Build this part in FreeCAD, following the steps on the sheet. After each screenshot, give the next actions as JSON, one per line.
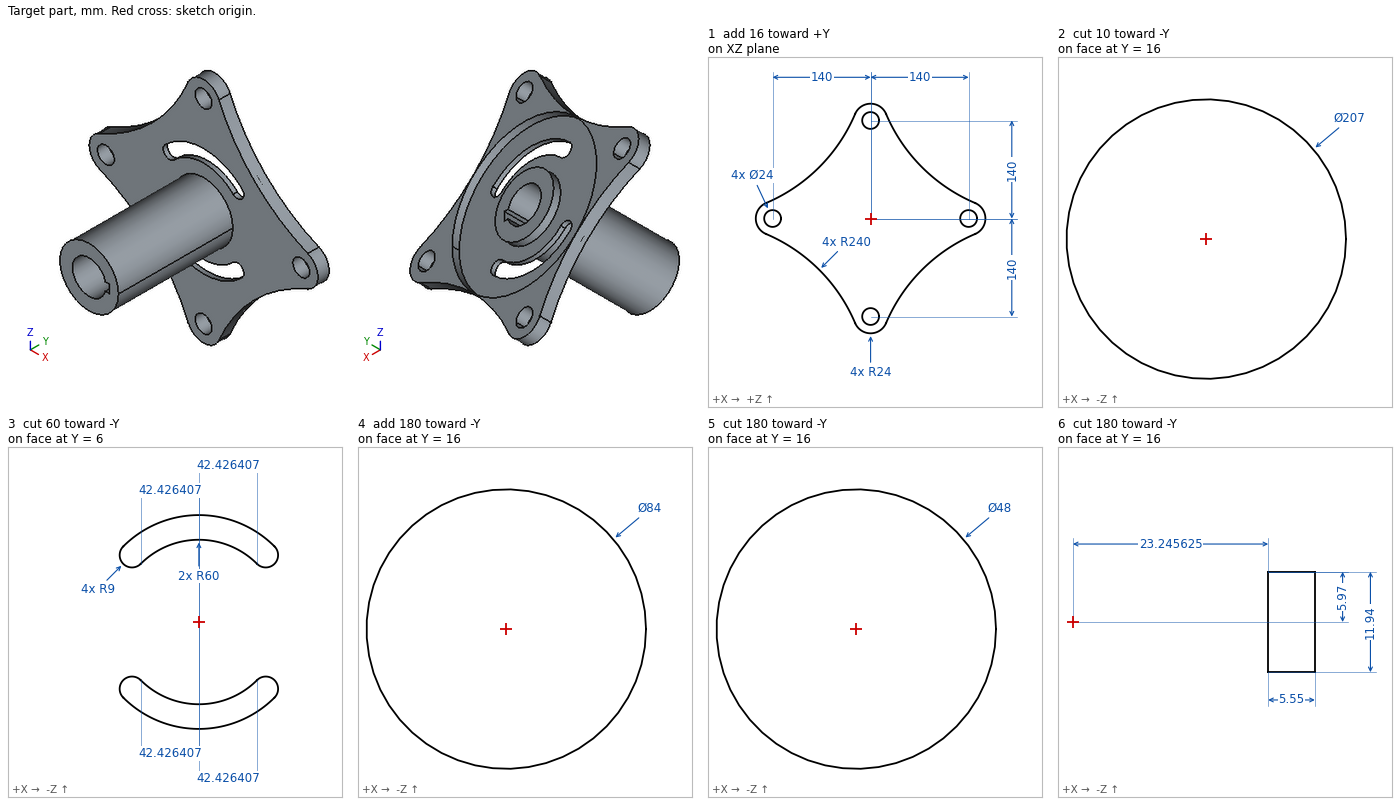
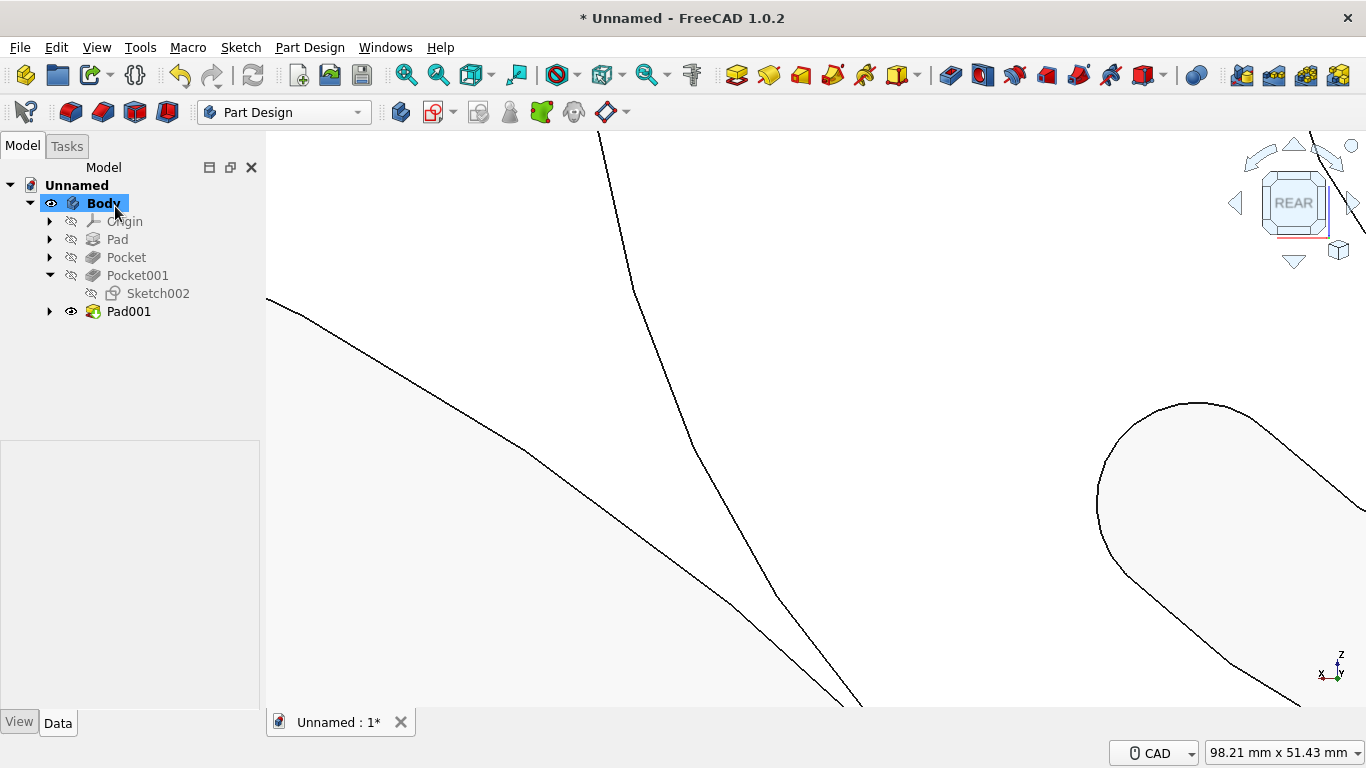
{"action": "left_click", "coordinate": [408, 76]}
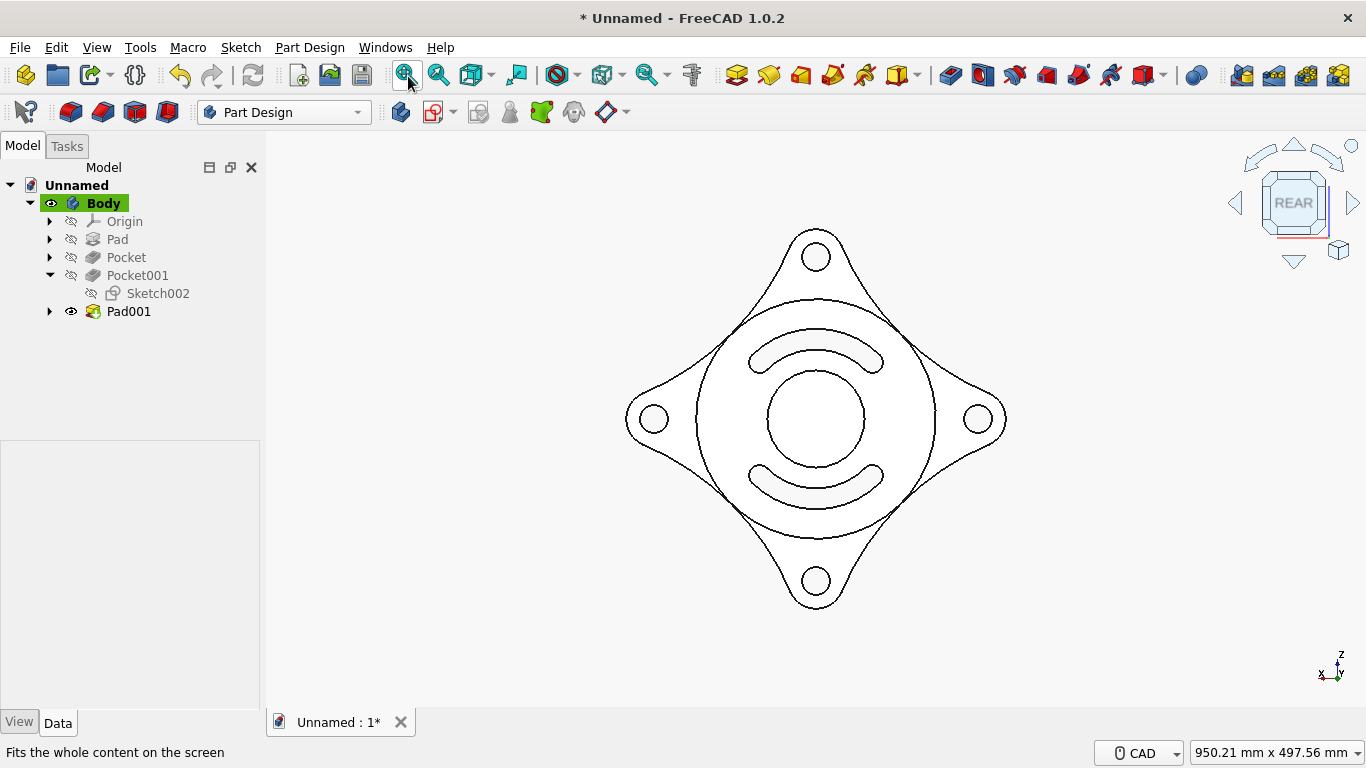
{"action": "scroll", "coordinate": [708, 472], "scroll_direction": "up", "scroll_amount": 11}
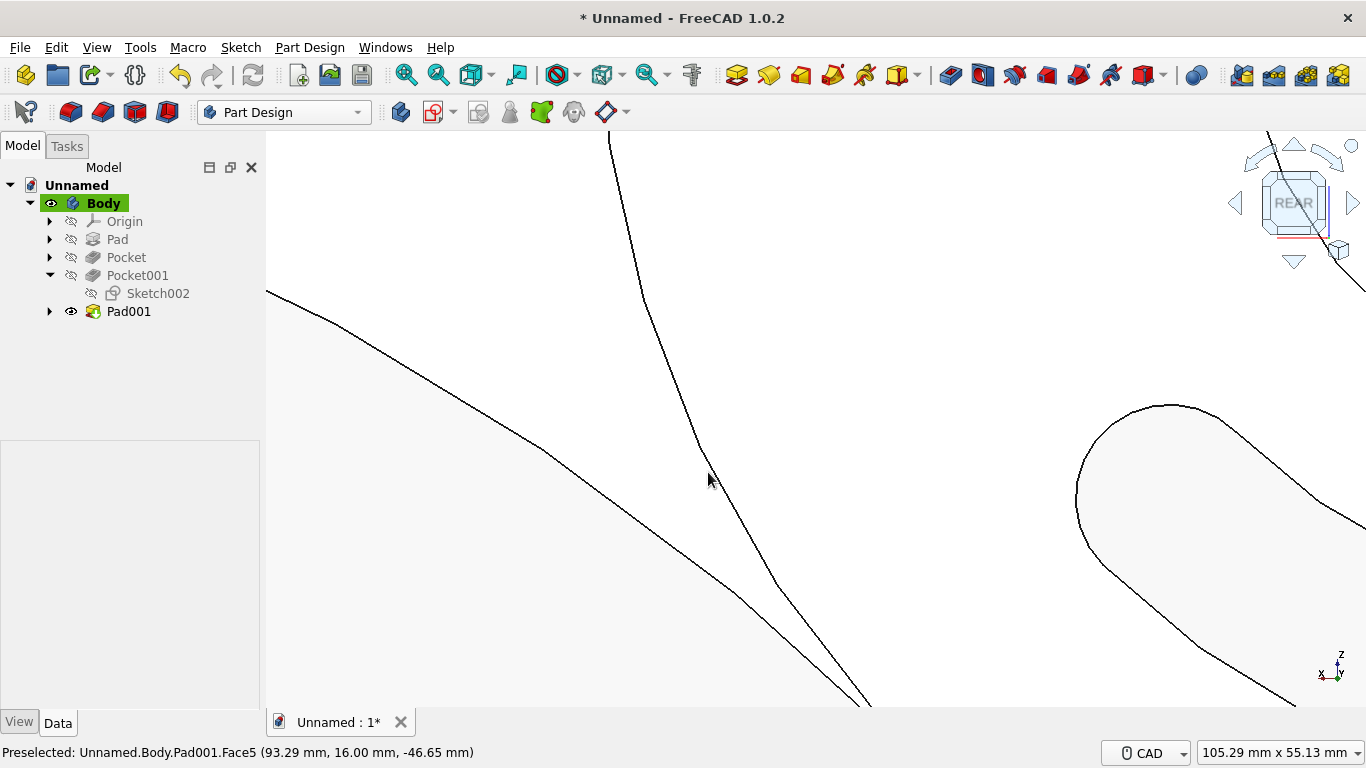
{"action": "left_click", "coordinate": [700, 477]}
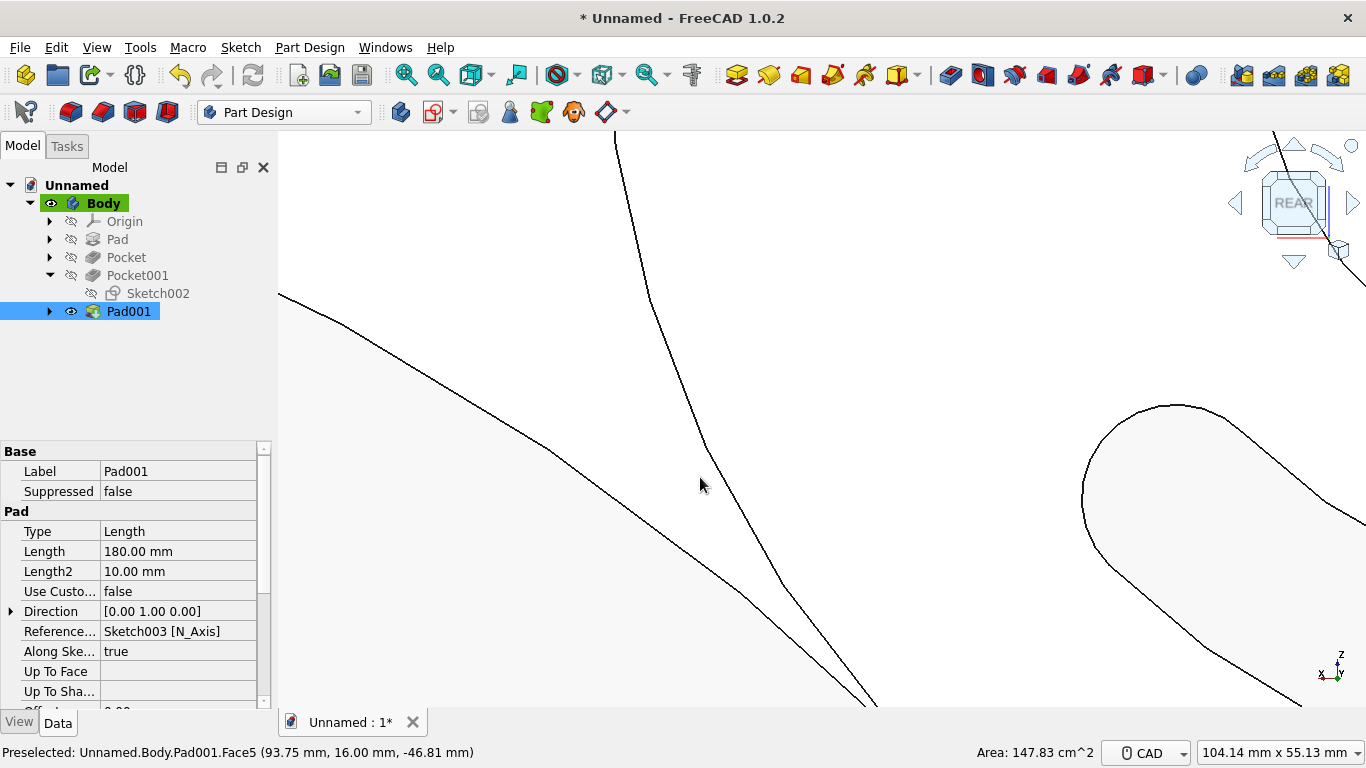
{"action": "left_click", "coordinate": [434, 112]}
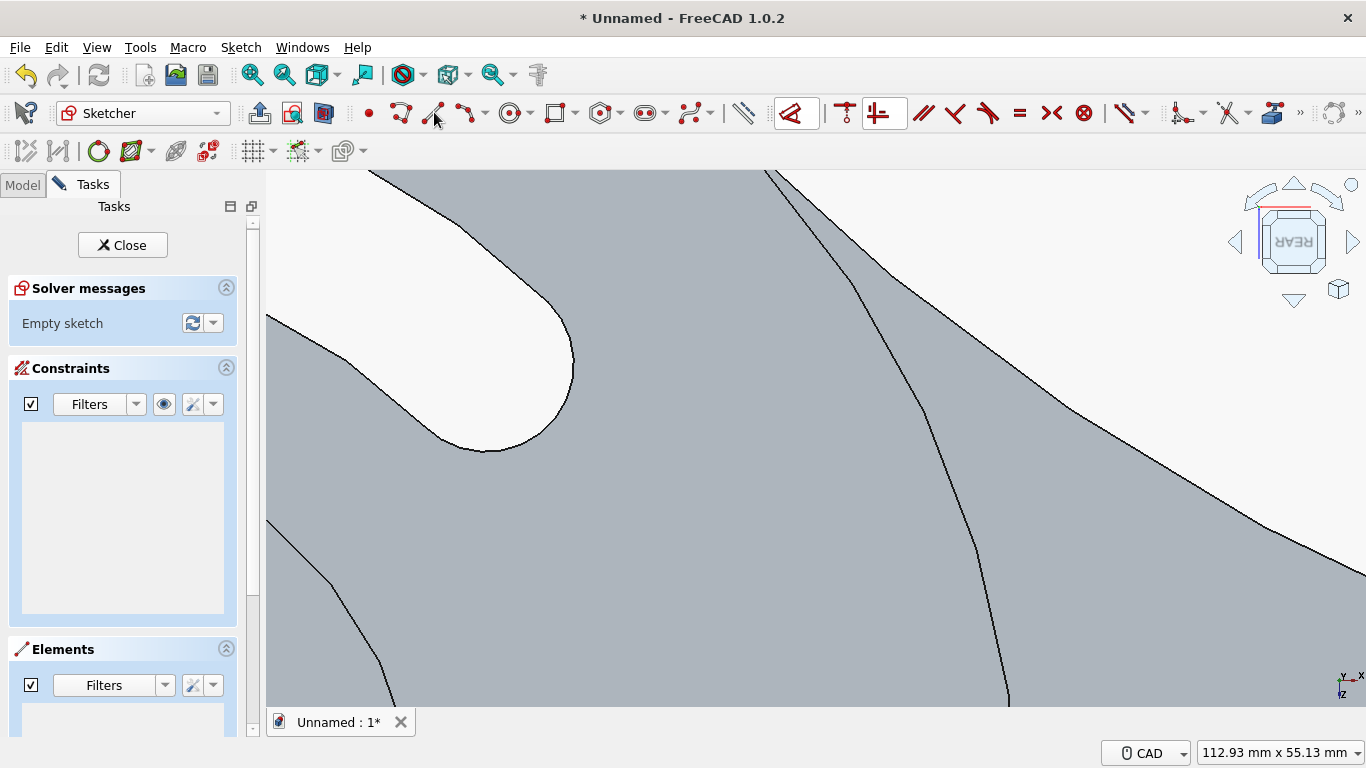
{"action": "scroll", "coordinate": [1201, 198], "scroll_direction": "down", "scroll_amount": 4}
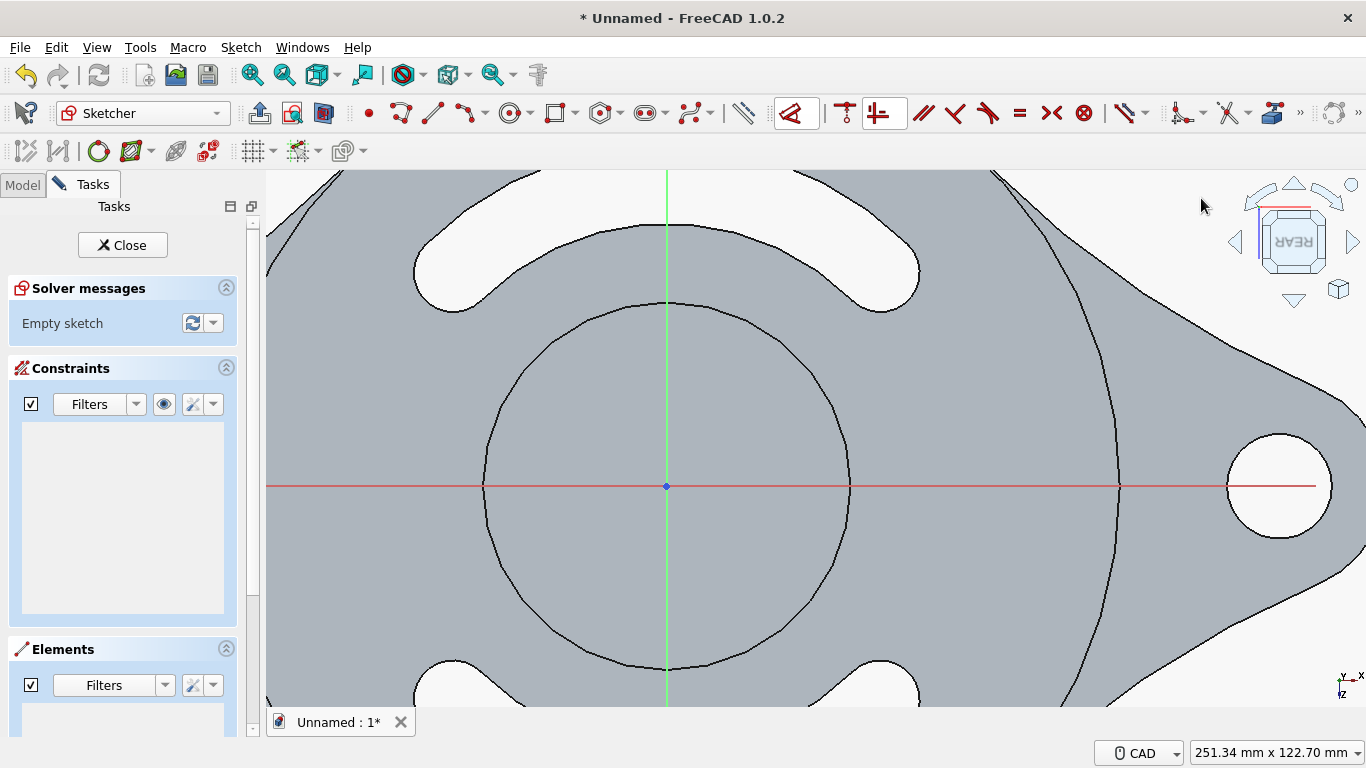
{"action": "scroll", "coordinate": [503, 583], "scroll_direction": "up", "scroll_amount": 2}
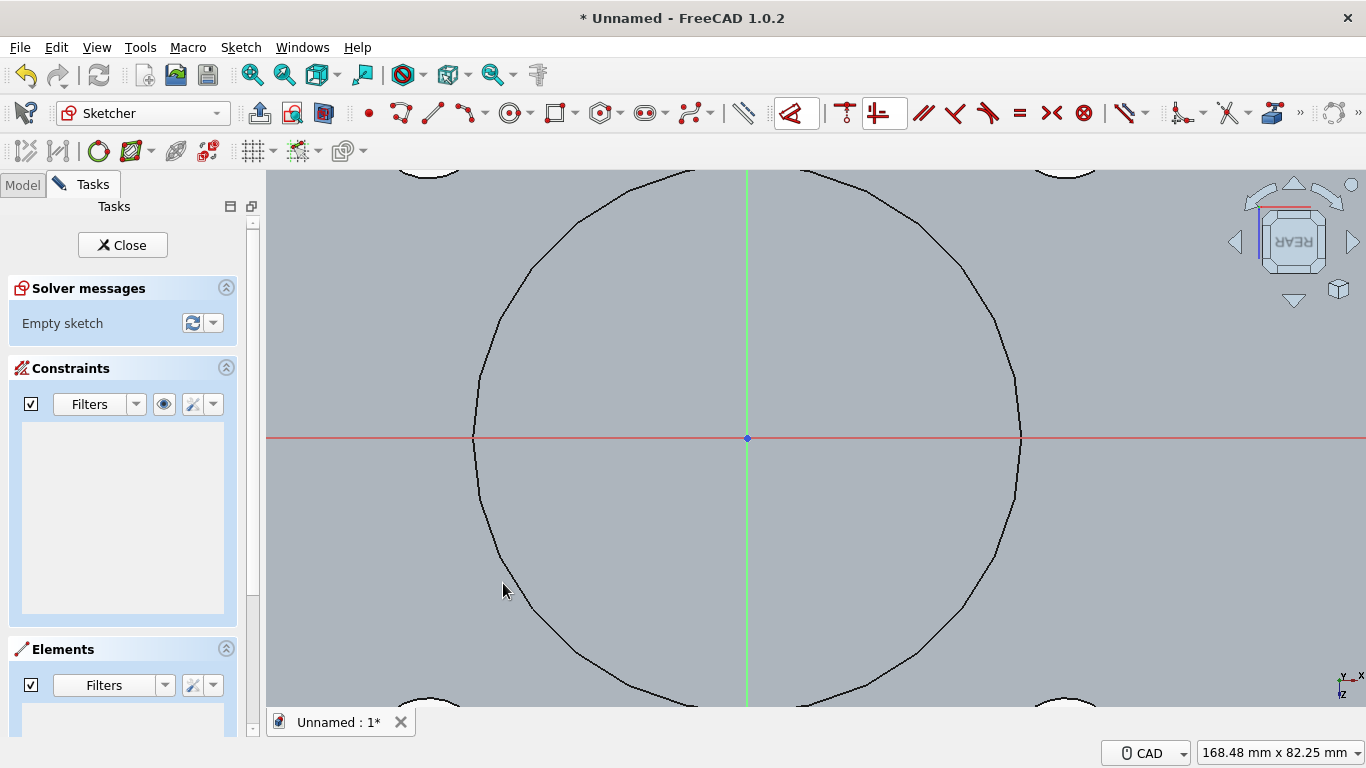
{"action": "left_click", "coordinate": [510, 114]}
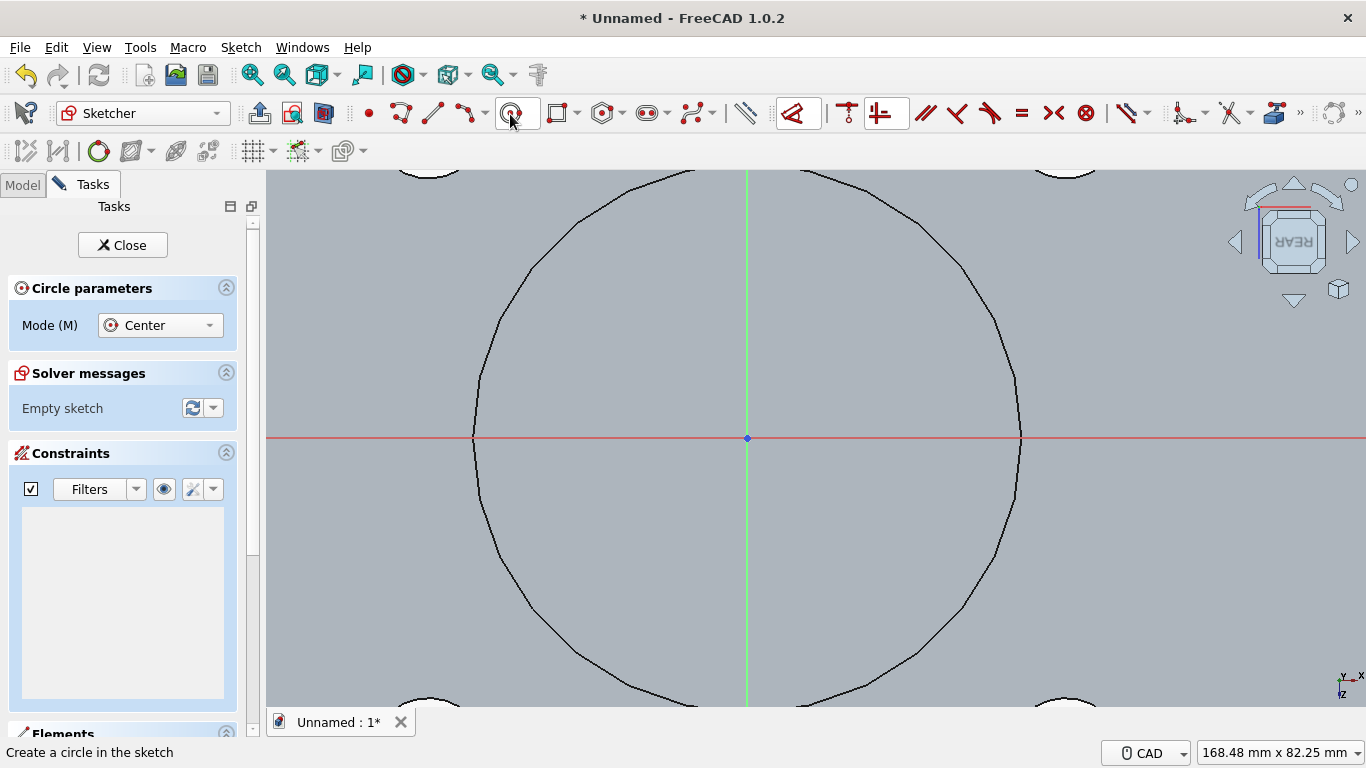
{"action": "left_click", "coordinate": [747, 438]}
{"action": "left_click", "coordinate": [858, 327]}
{"action": "key", "text": "Escape"}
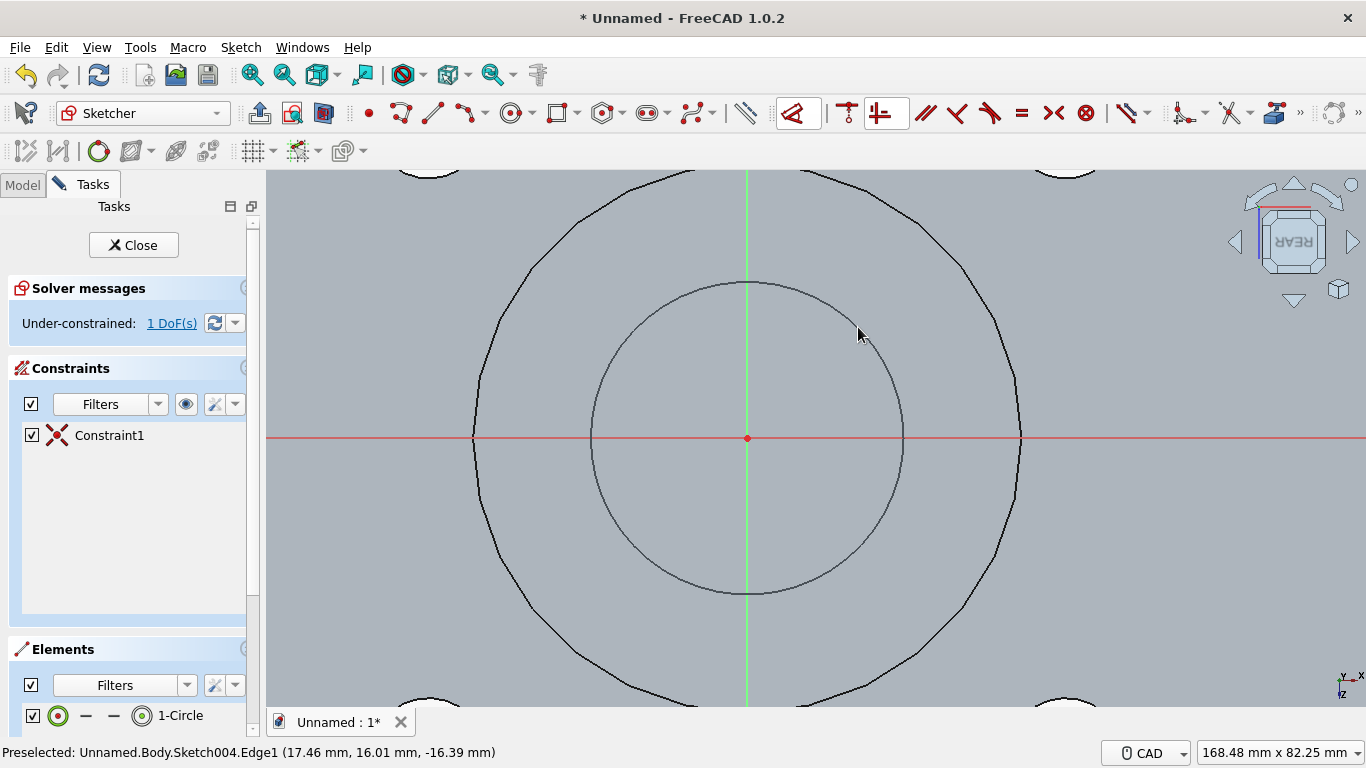
{"action": "left_click", "coordinate": [857, 327]}